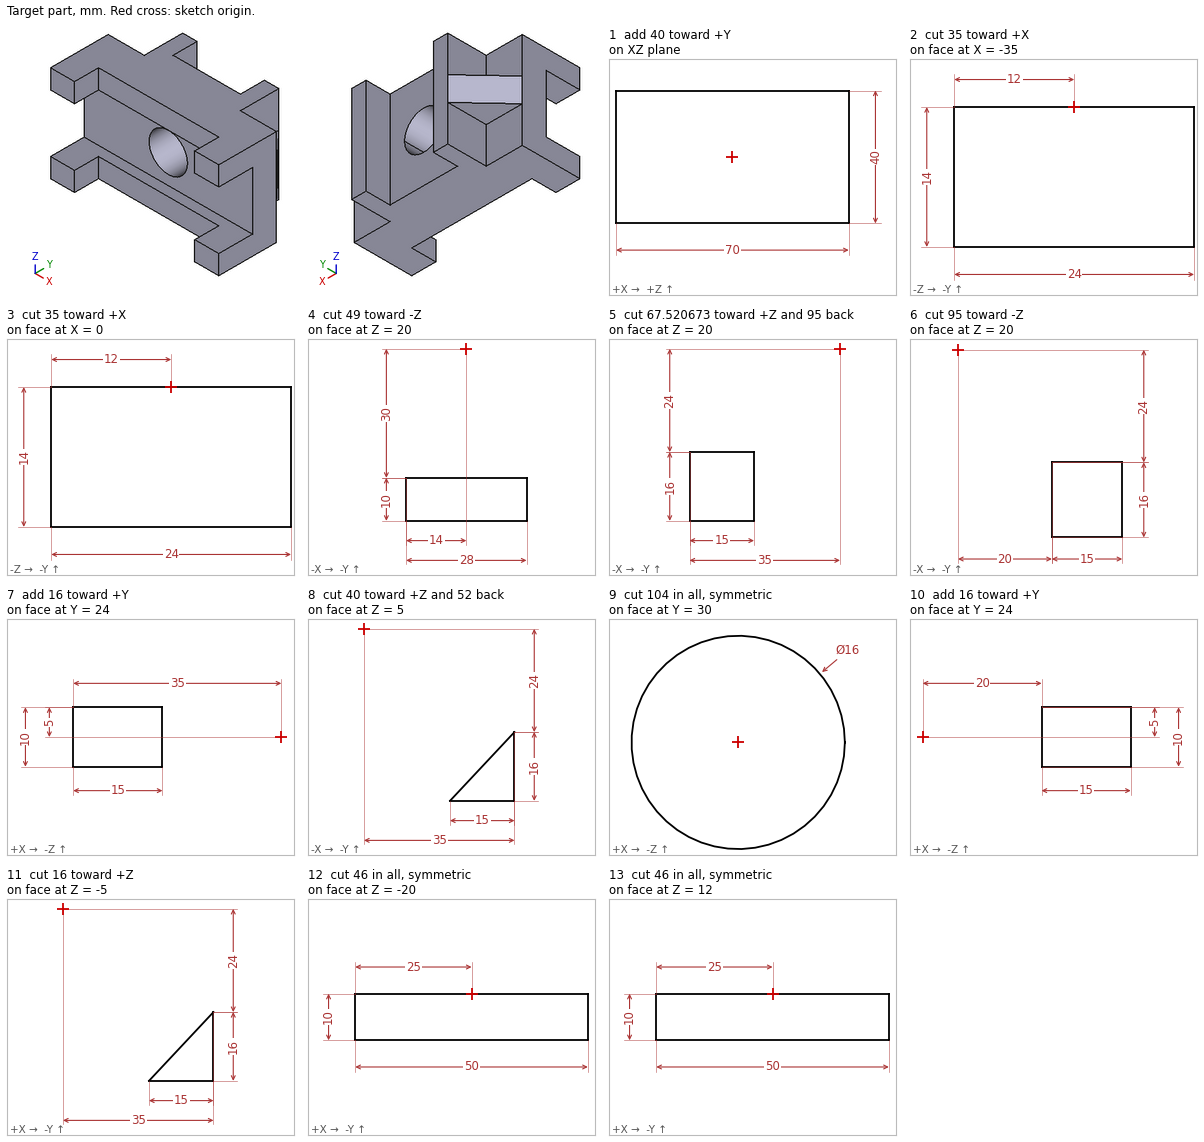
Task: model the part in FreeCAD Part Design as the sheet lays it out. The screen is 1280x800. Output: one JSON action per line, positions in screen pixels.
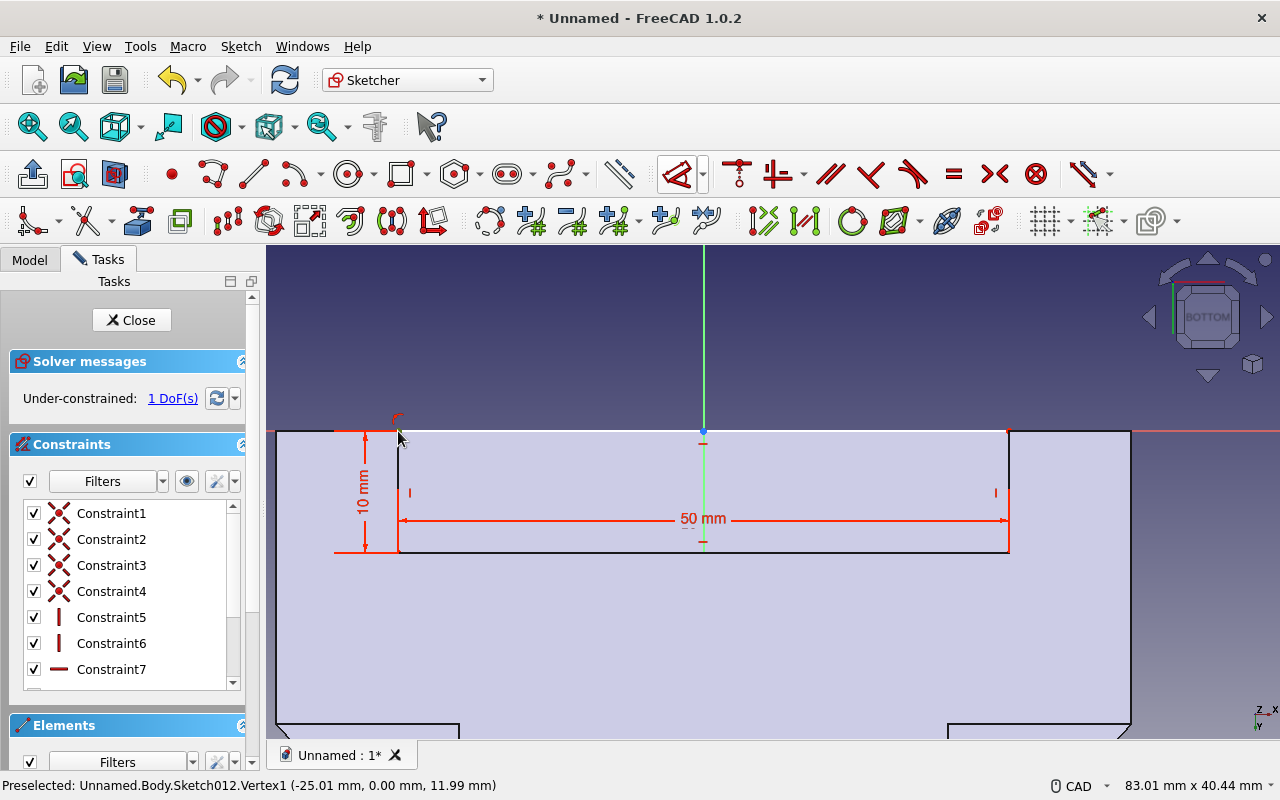
{"action": "key", "text": "l"}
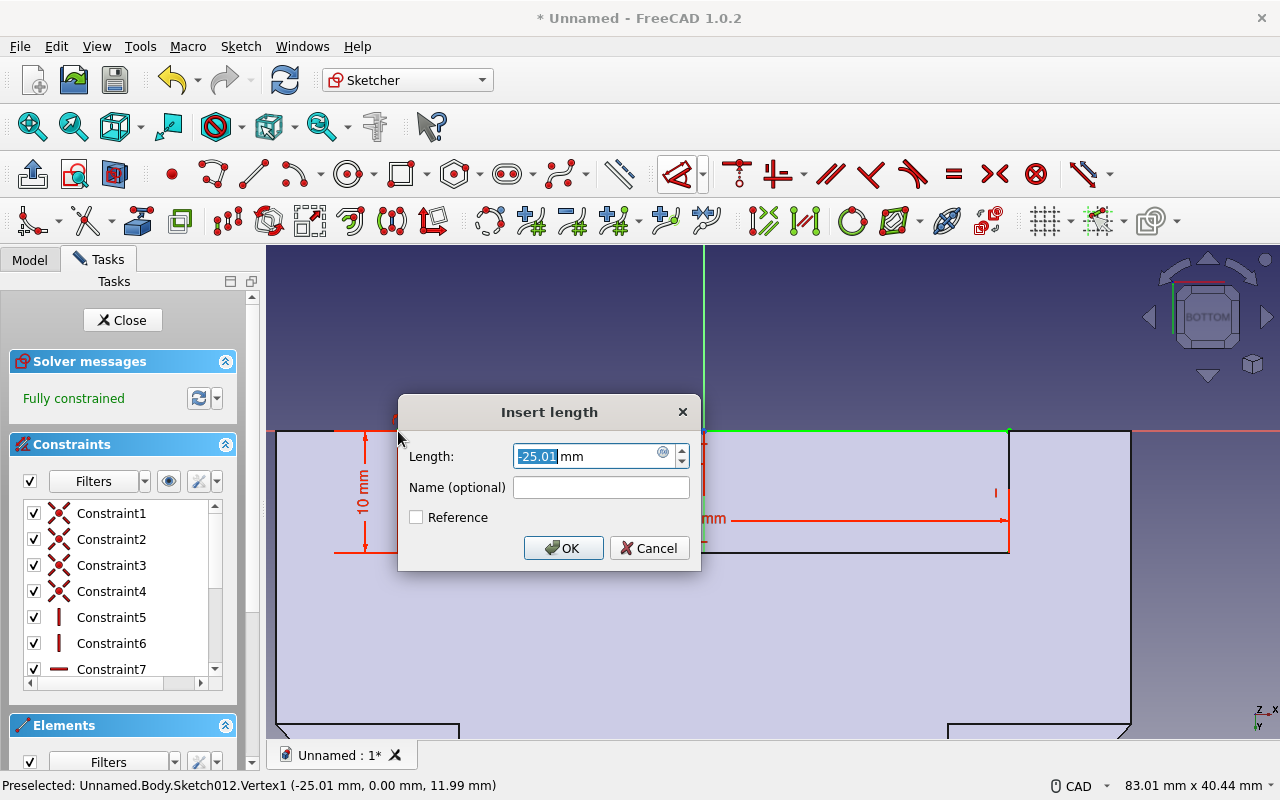
{"action": "type", "text": "-25"}
{"action": "key", "text": "Return"}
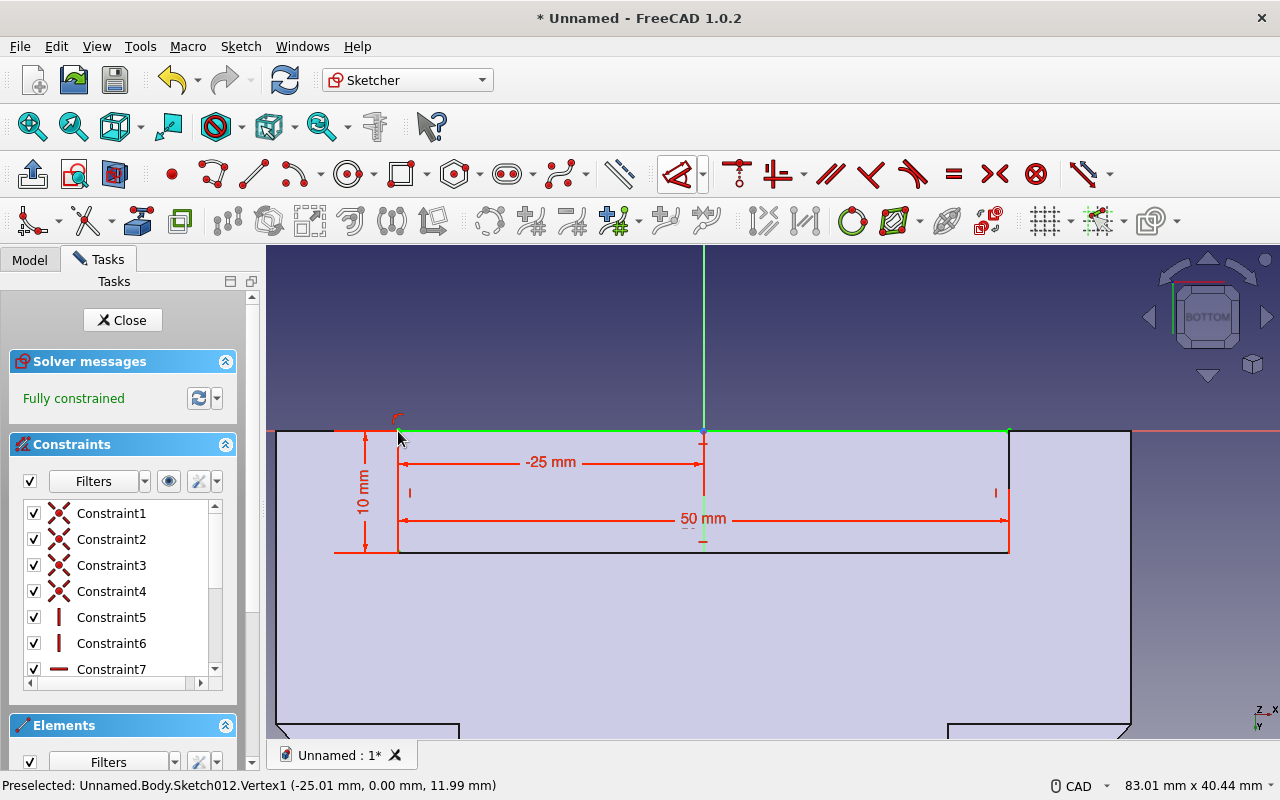
{"action": "left_click", "coordinate": [123, 320]}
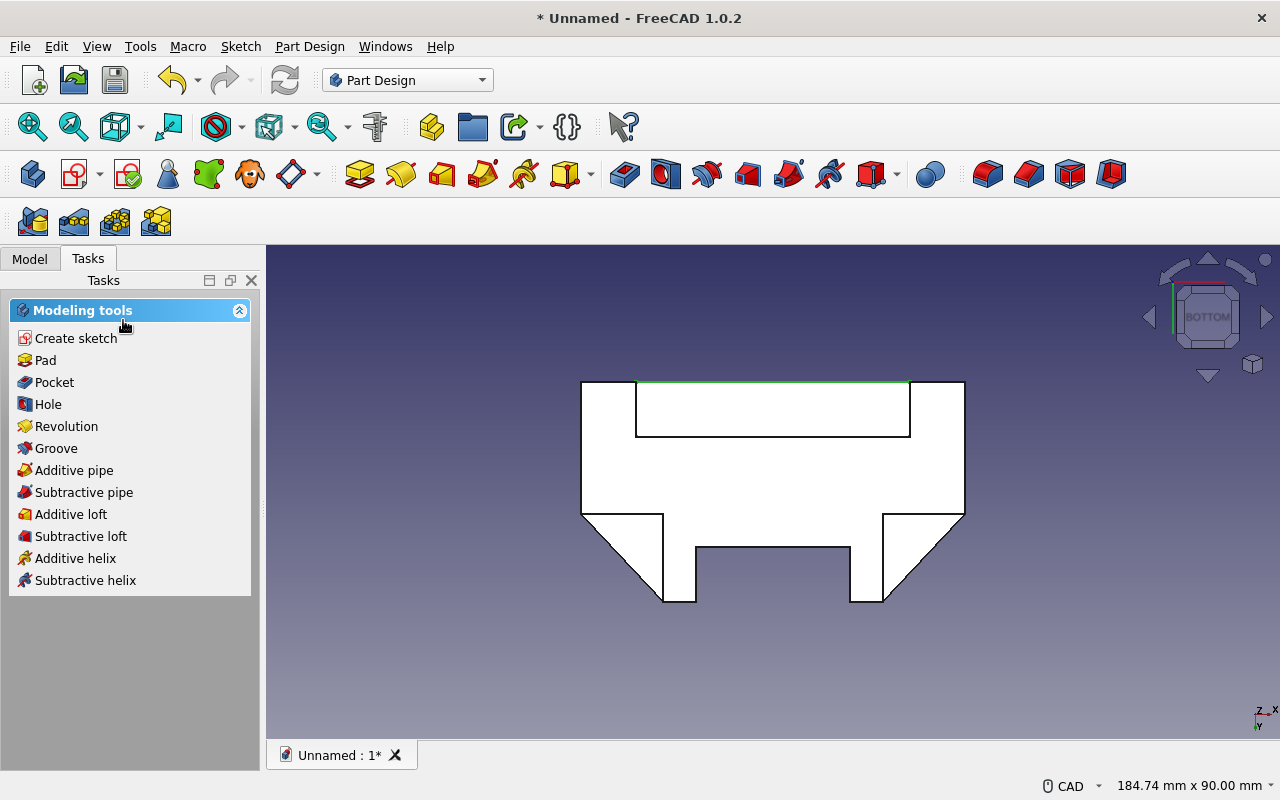
{"action": "left_click", "coordinate": [625, 174]}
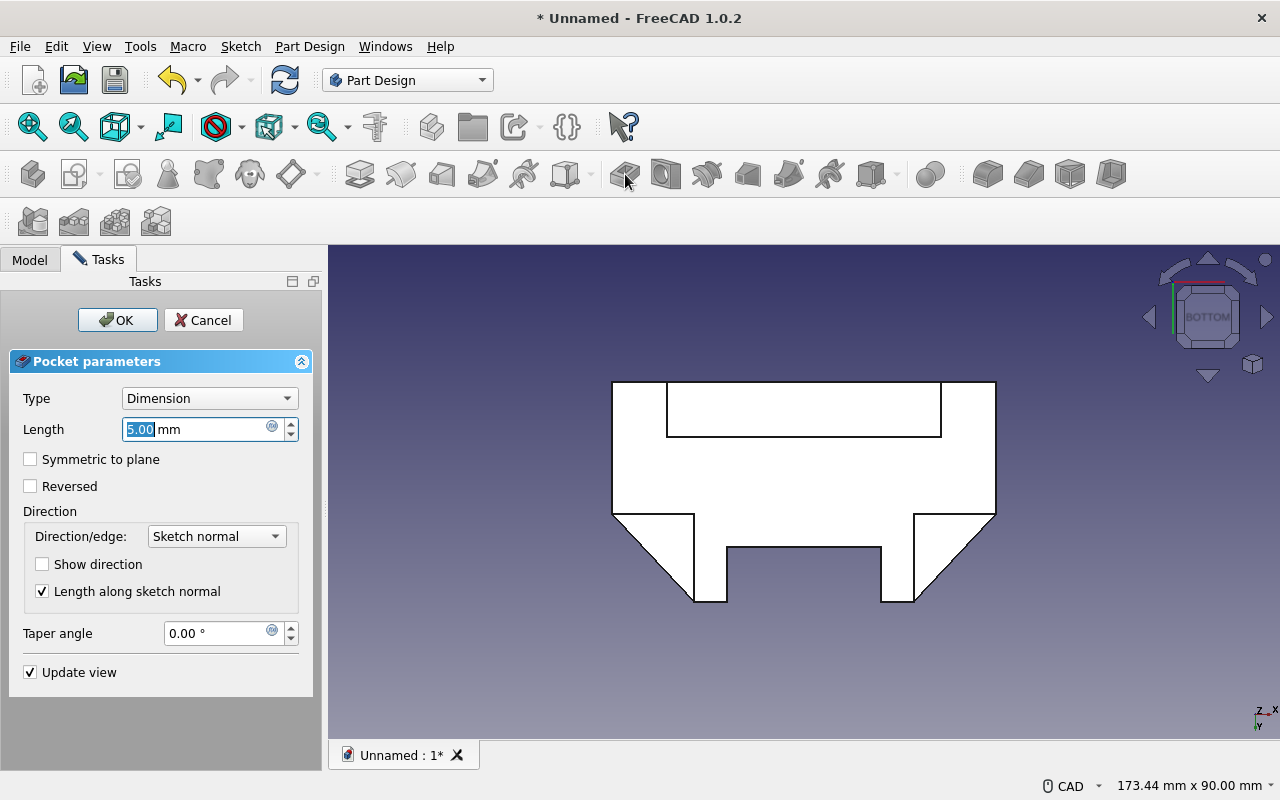
{"action": "type", "text": "46"}
{"action": "key", "text": "Tab"}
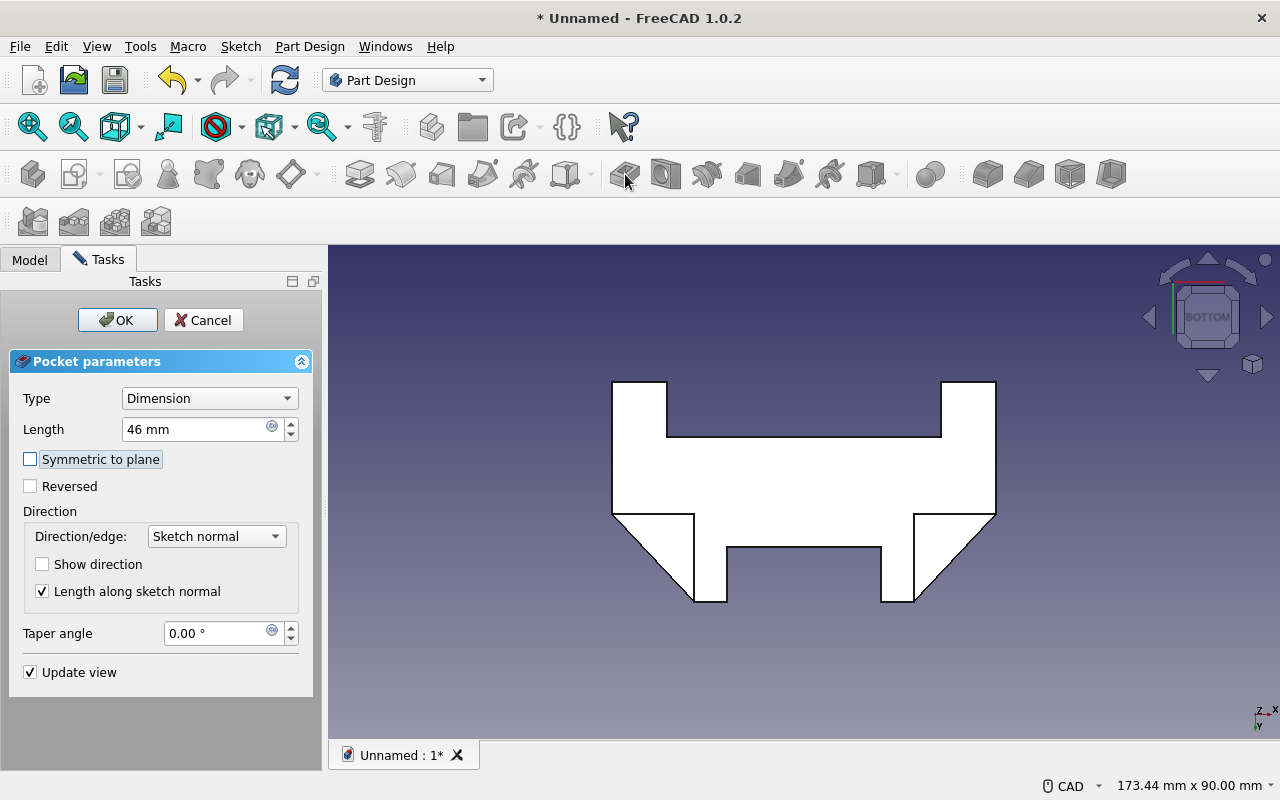
{"action": "left_click", "coordinate": [31, 459]}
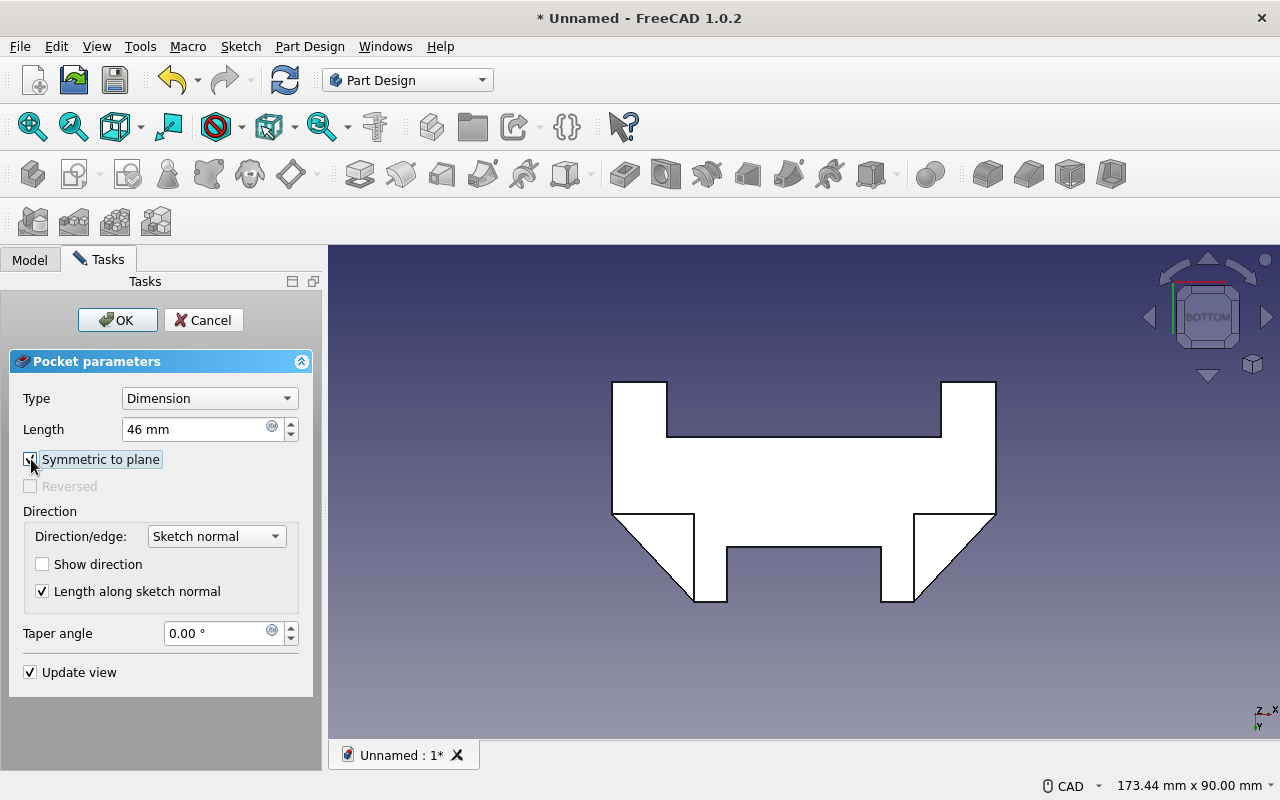
{"action": "left_click", "coordinate": [118, 320]}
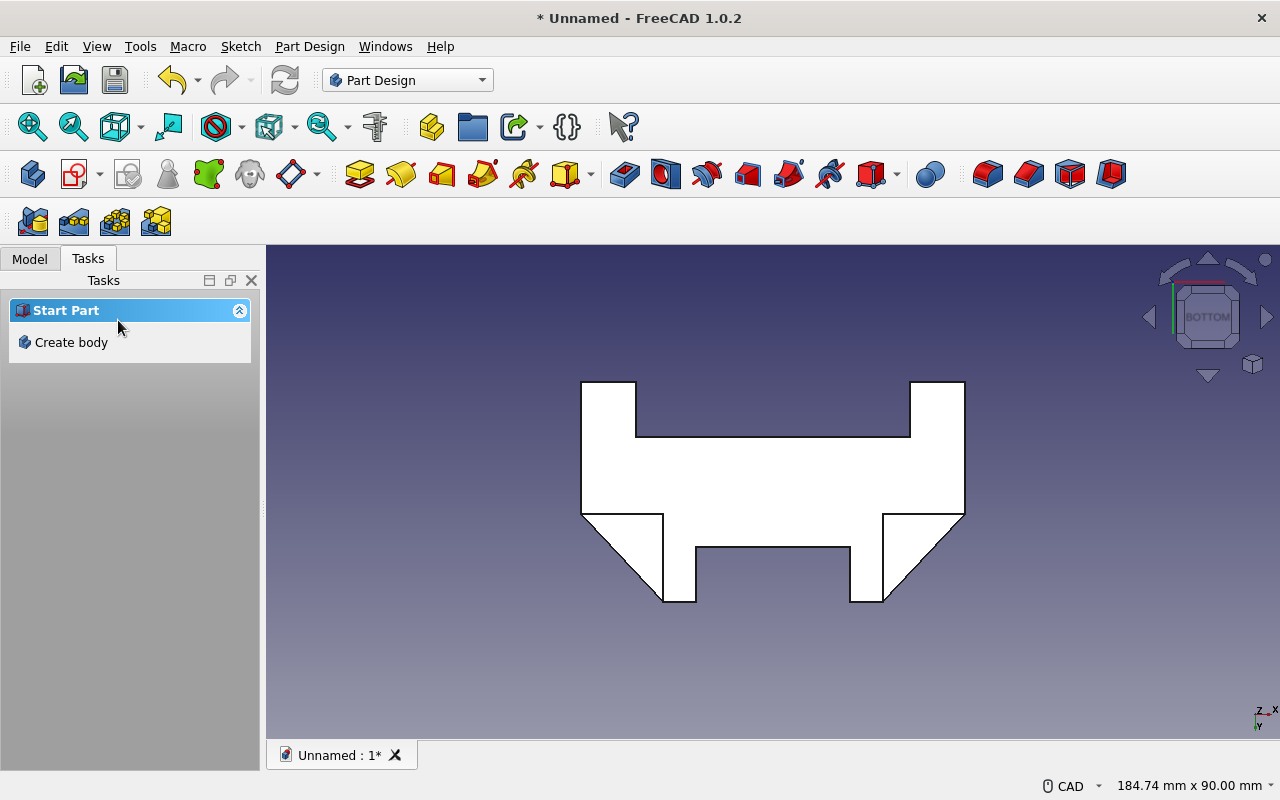
{"action": "key", "text": "0"}